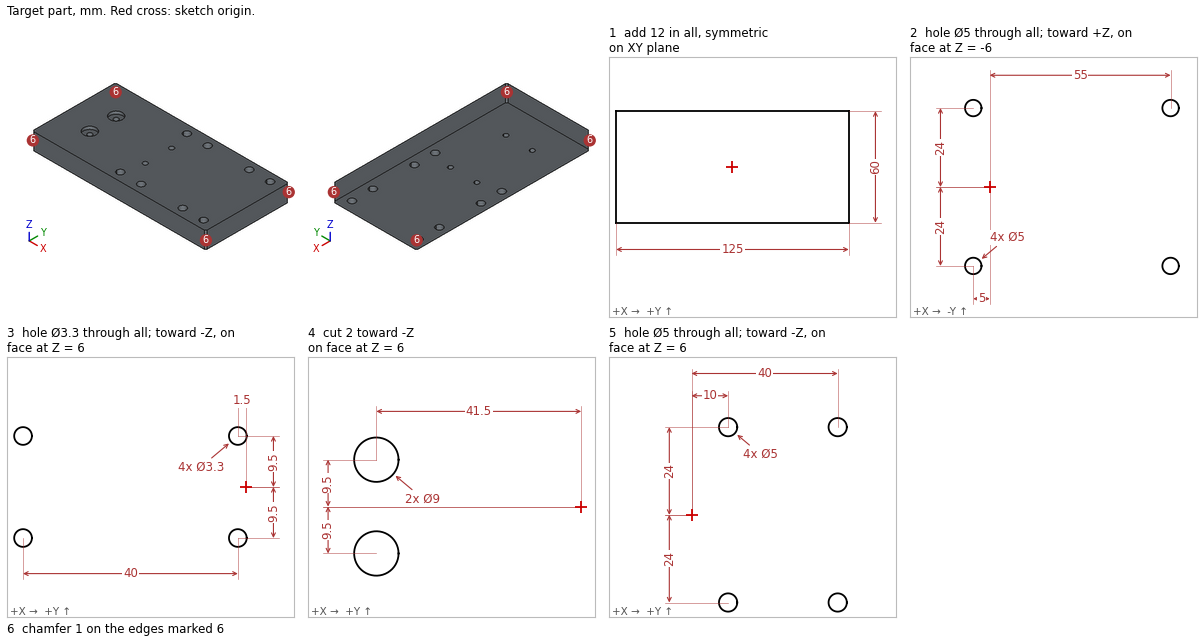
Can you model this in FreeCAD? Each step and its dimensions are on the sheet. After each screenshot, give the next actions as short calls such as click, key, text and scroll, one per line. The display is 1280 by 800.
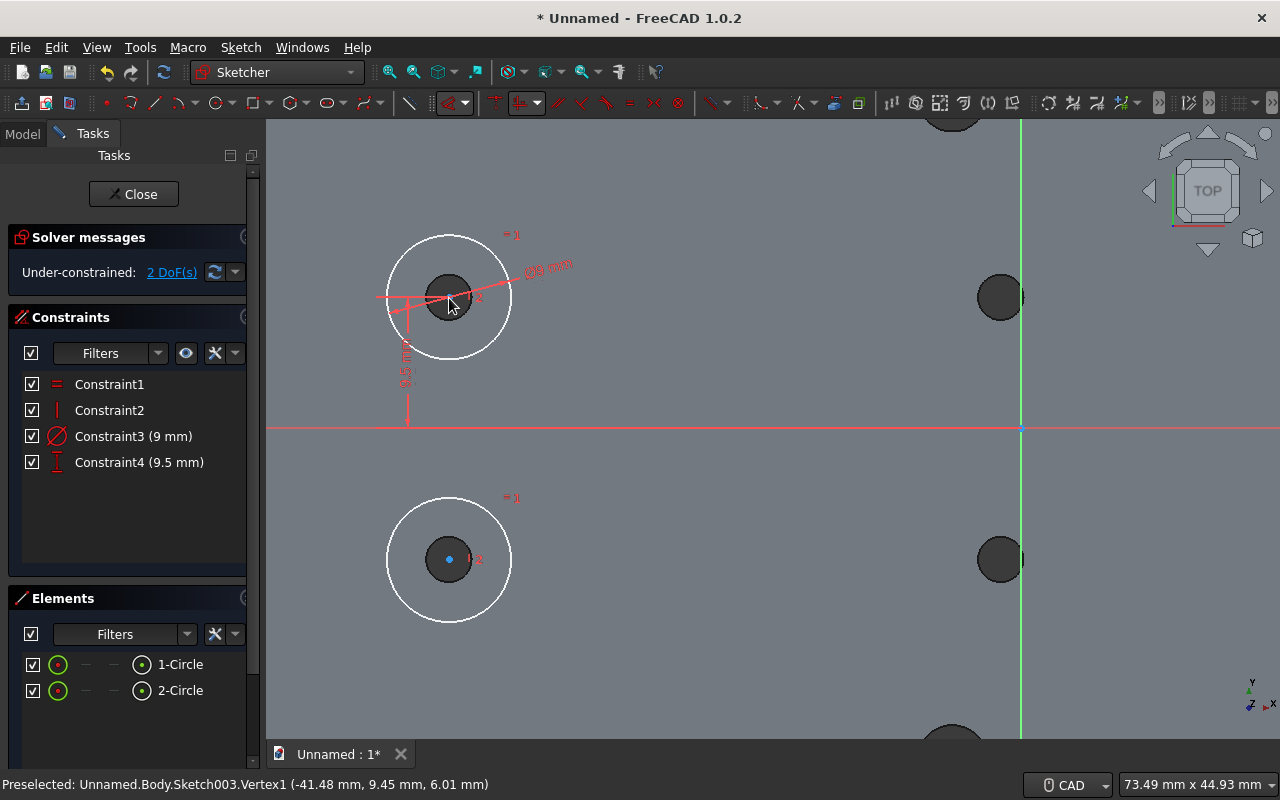
click(449, 560)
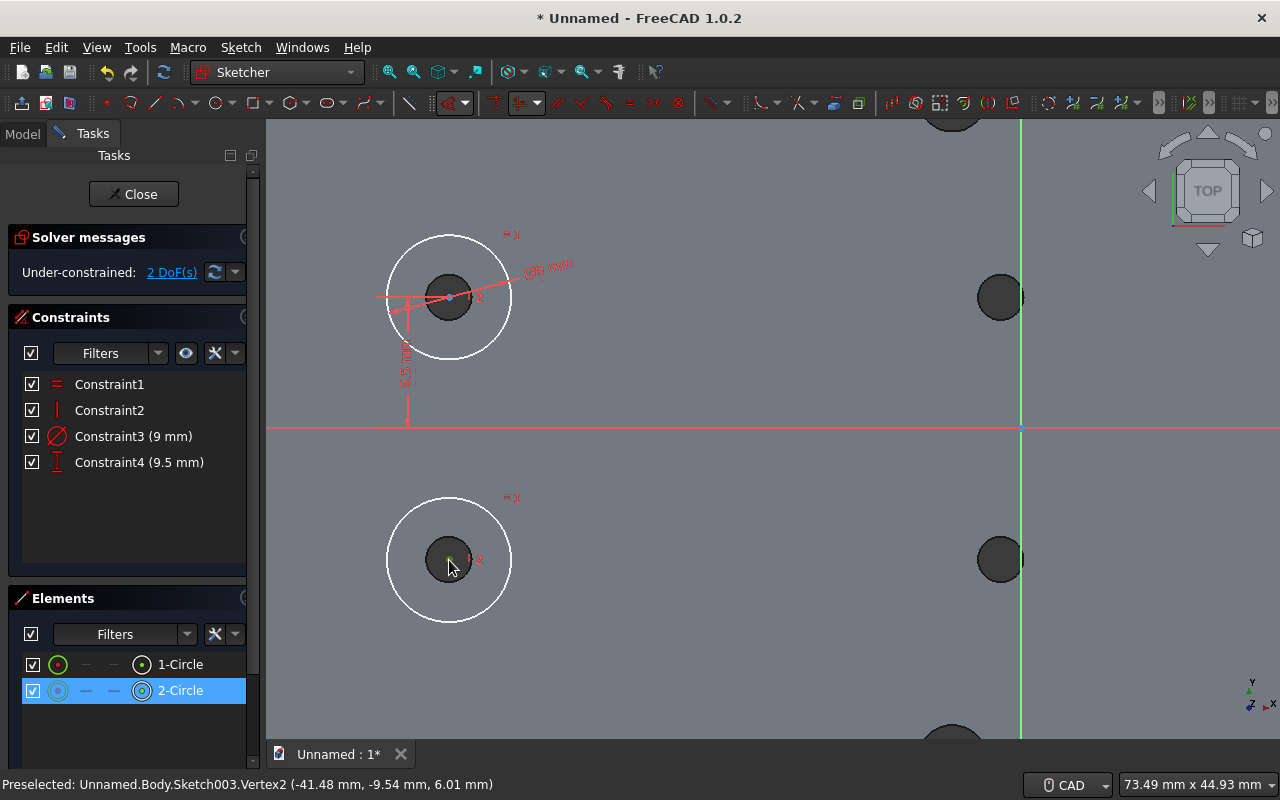
key(i)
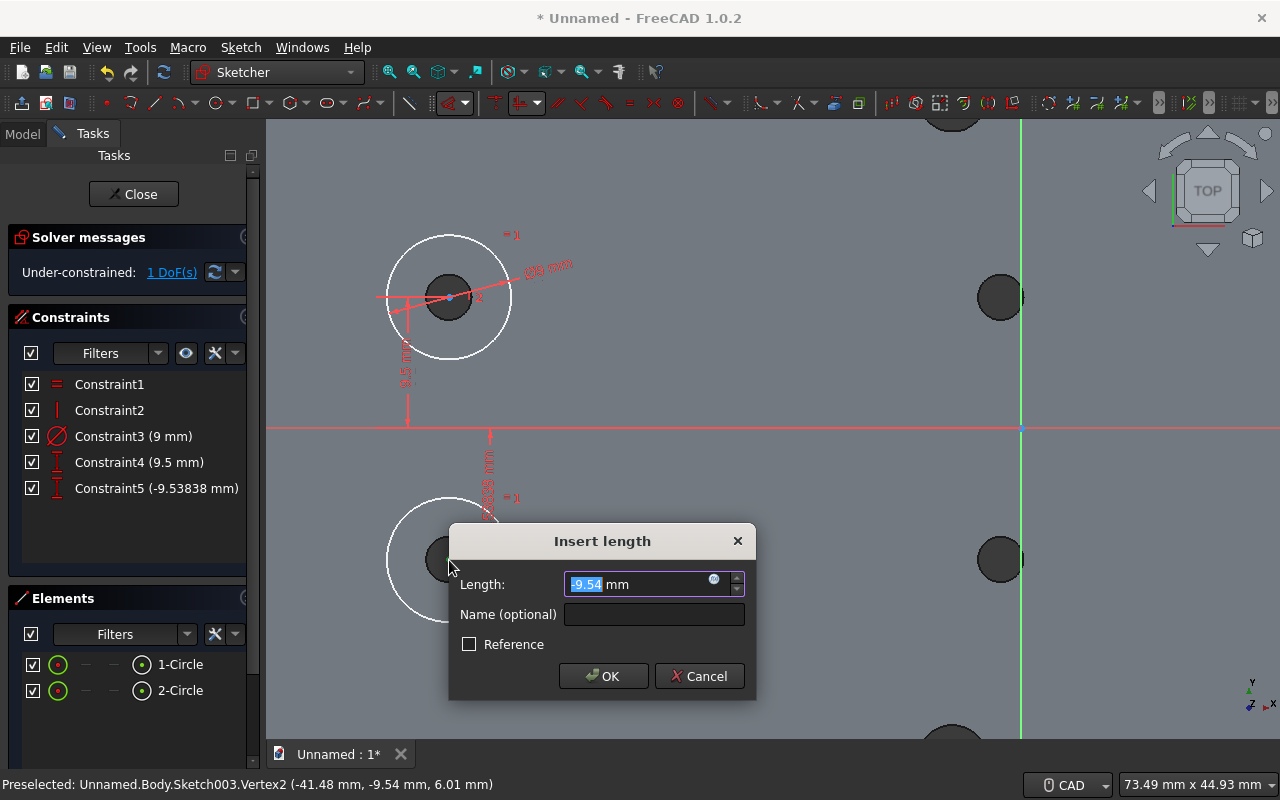
text(-9.5)
key(Return)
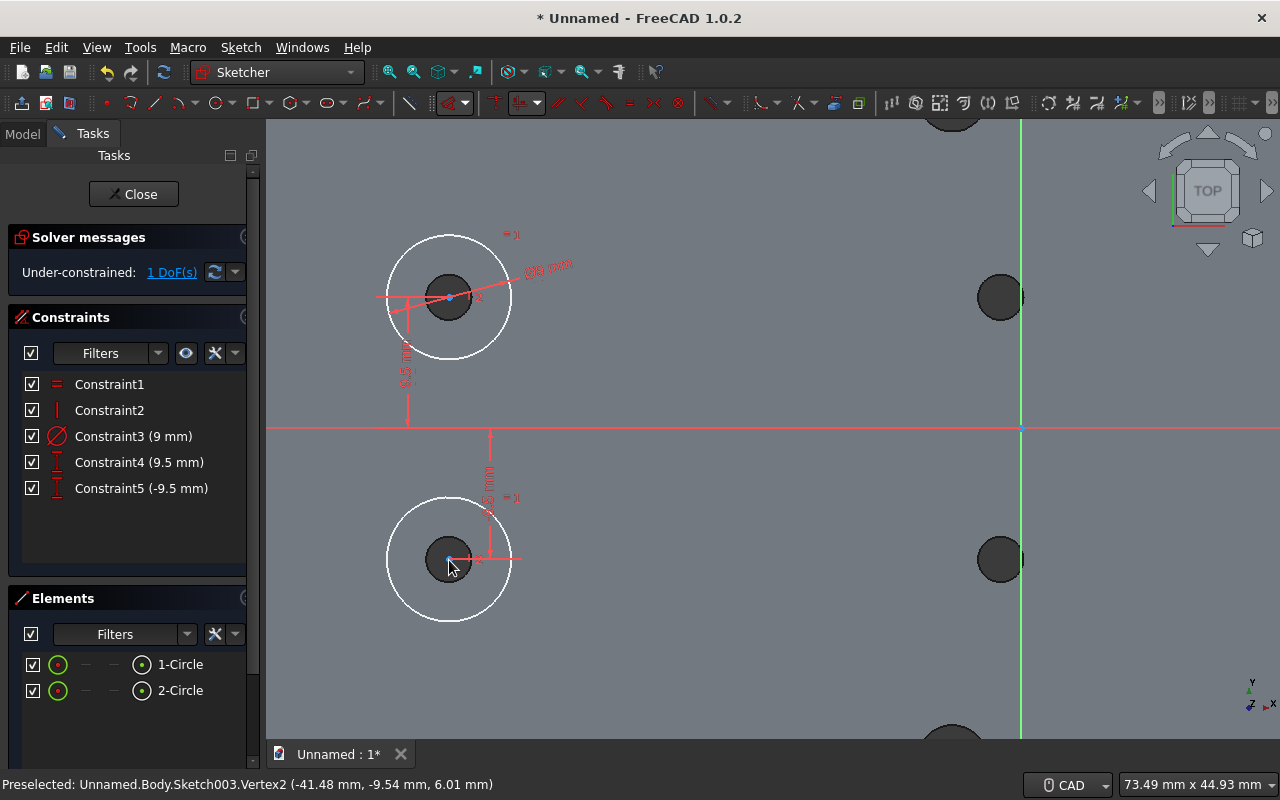
click(449, 297)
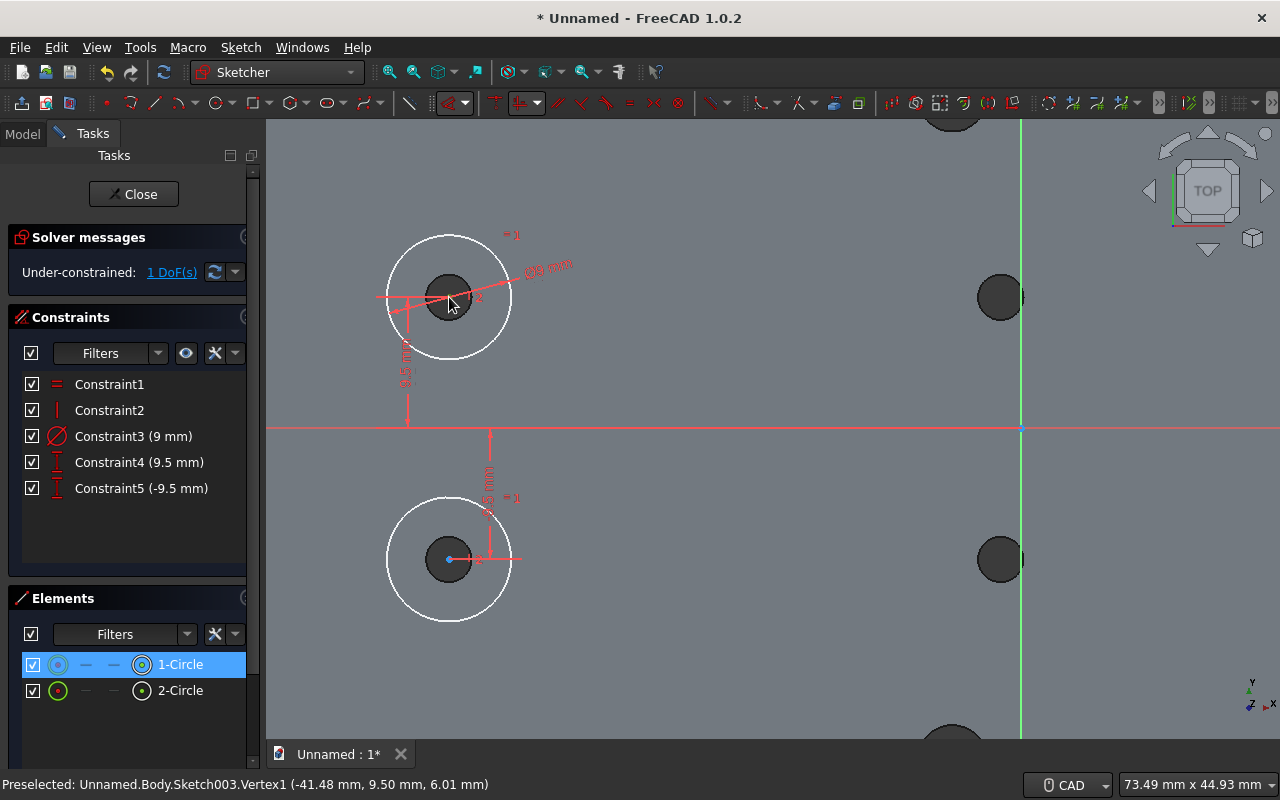
key(l)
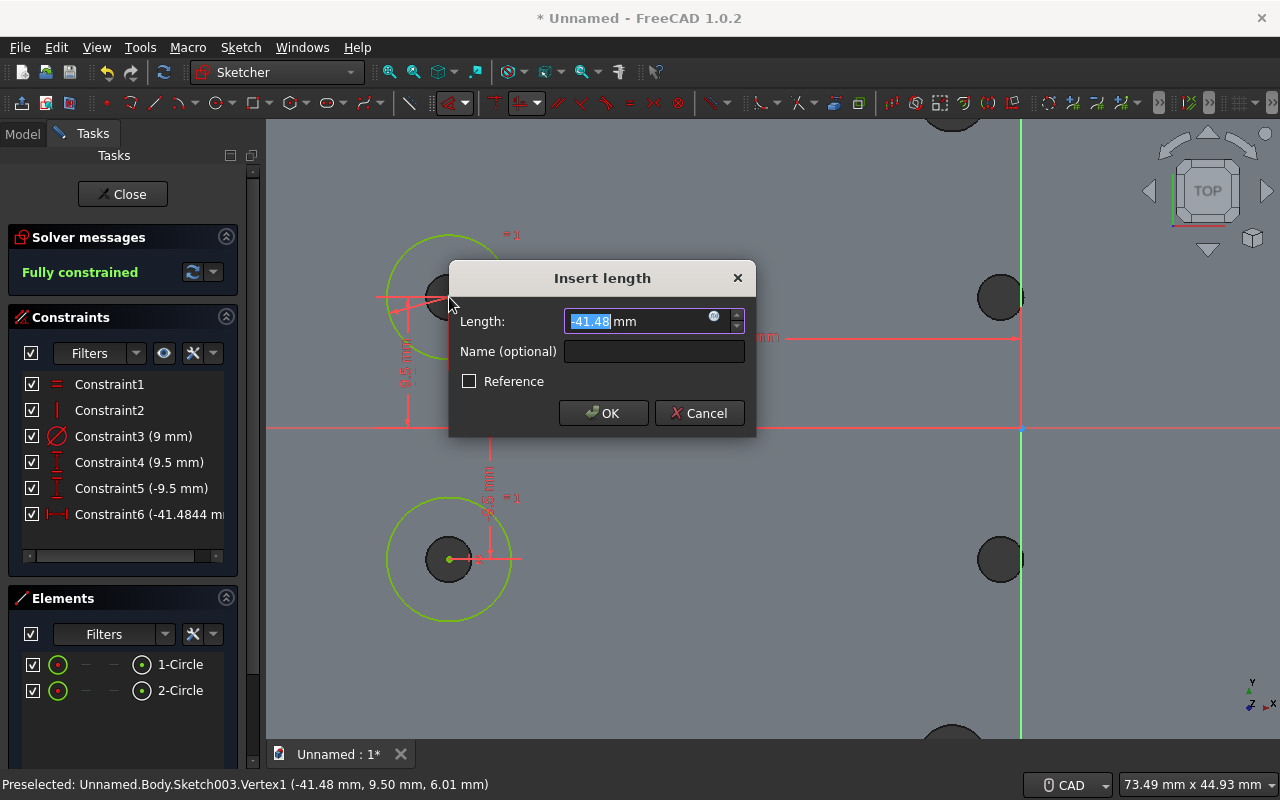
text(-41.5)
key(Return)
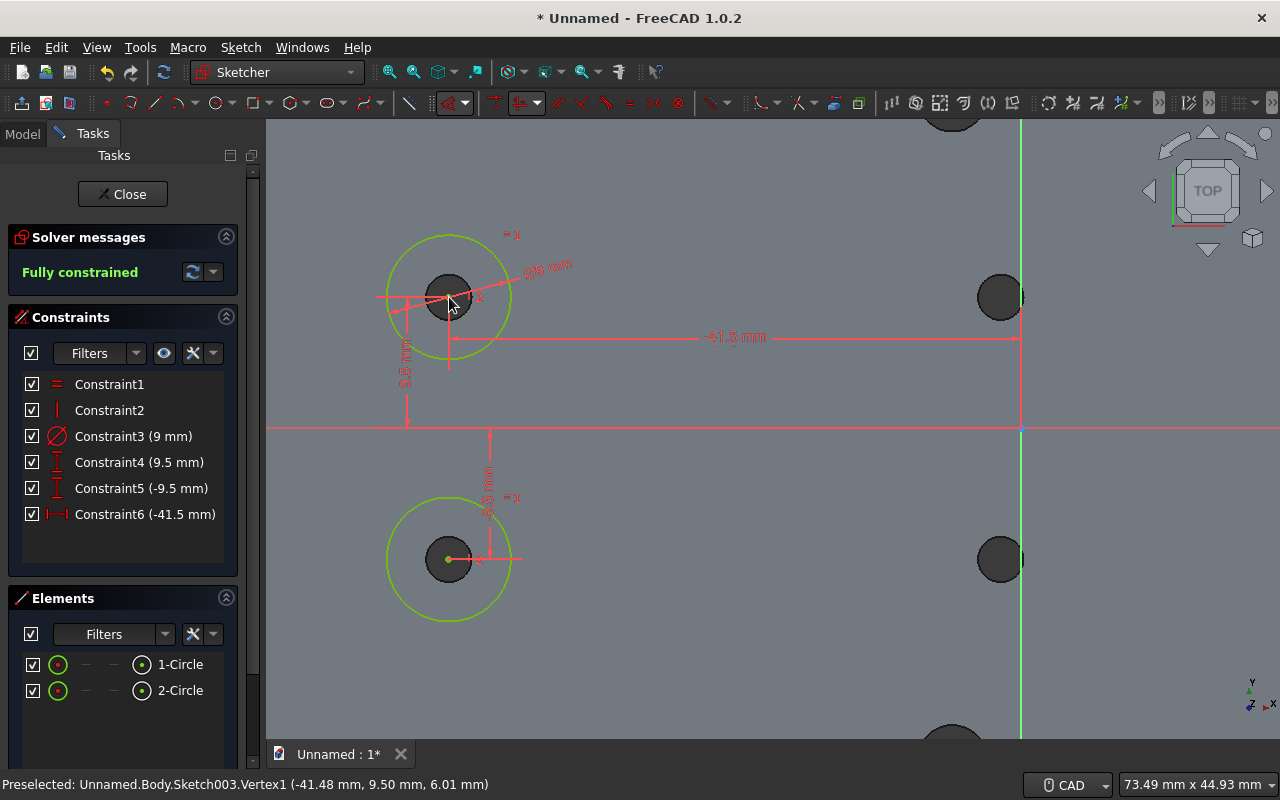
click(123, 194)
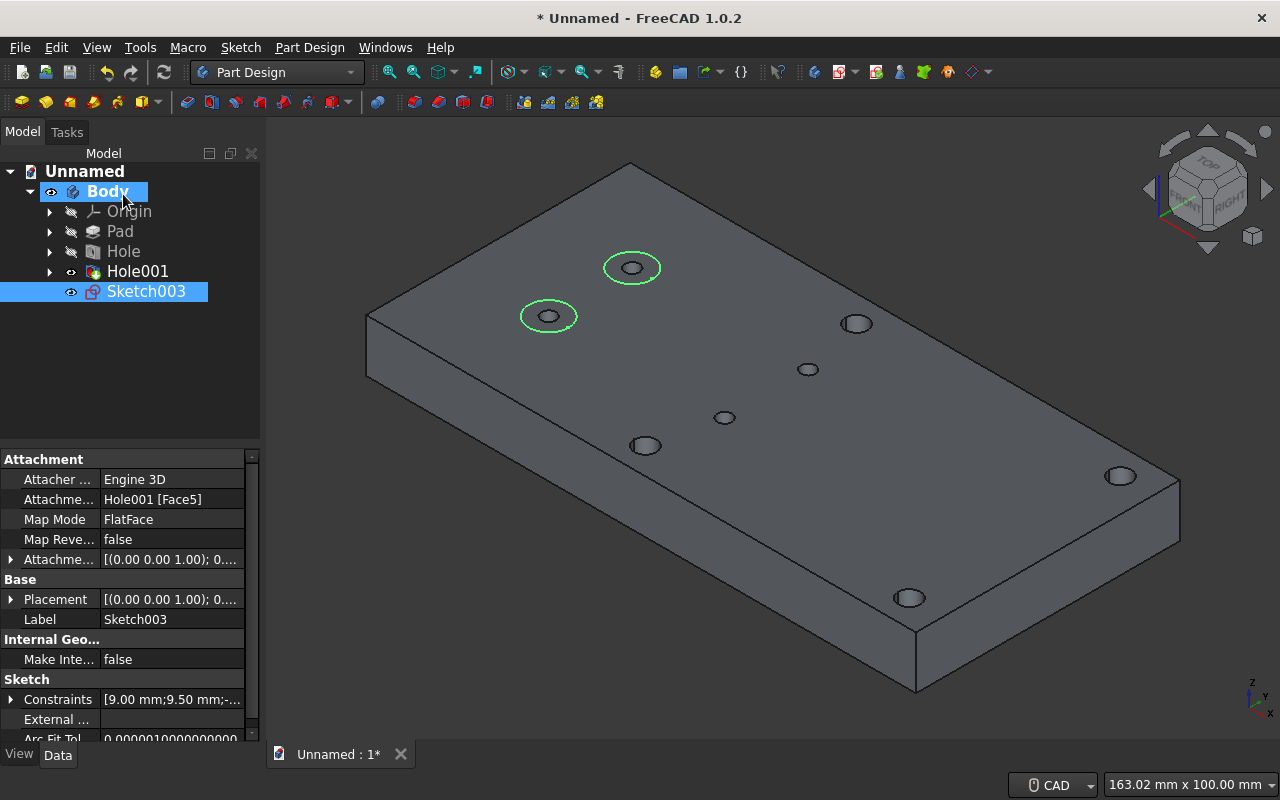
click(188, 102)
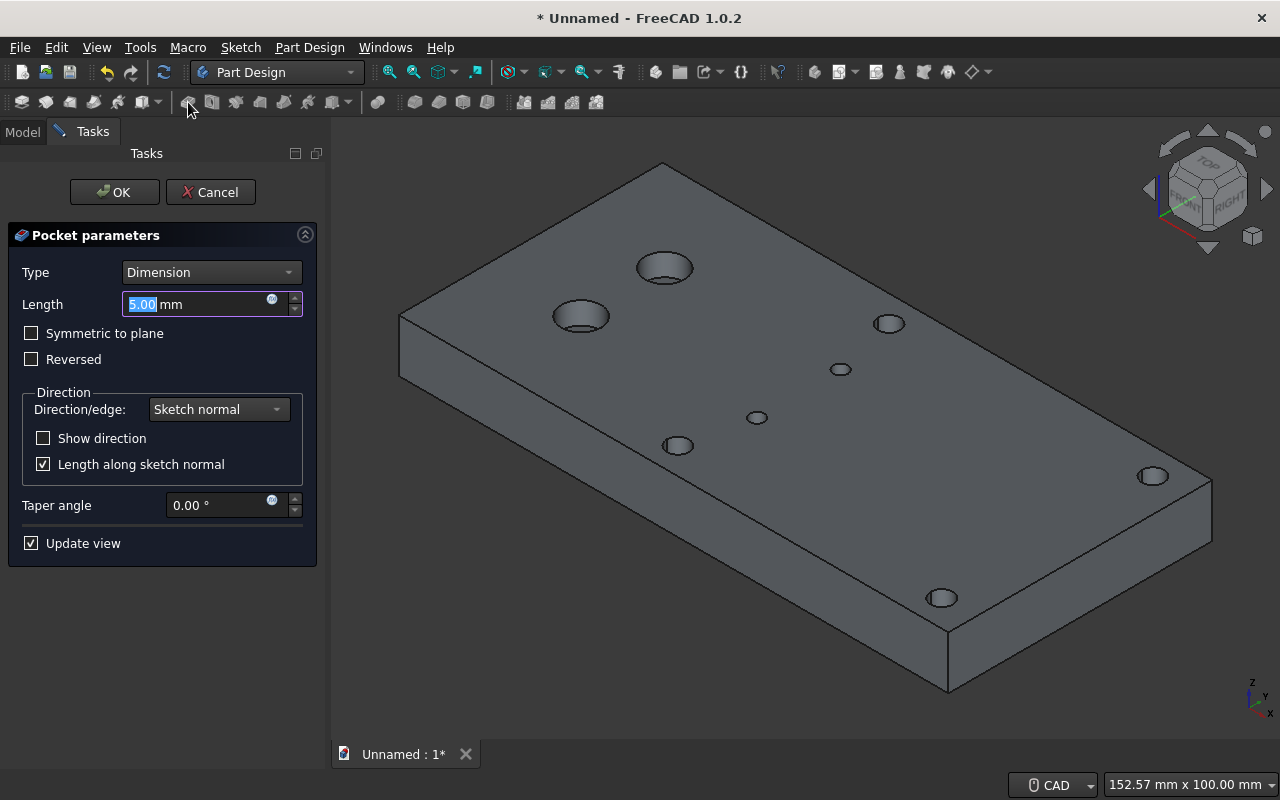
text(2)
key(Tab)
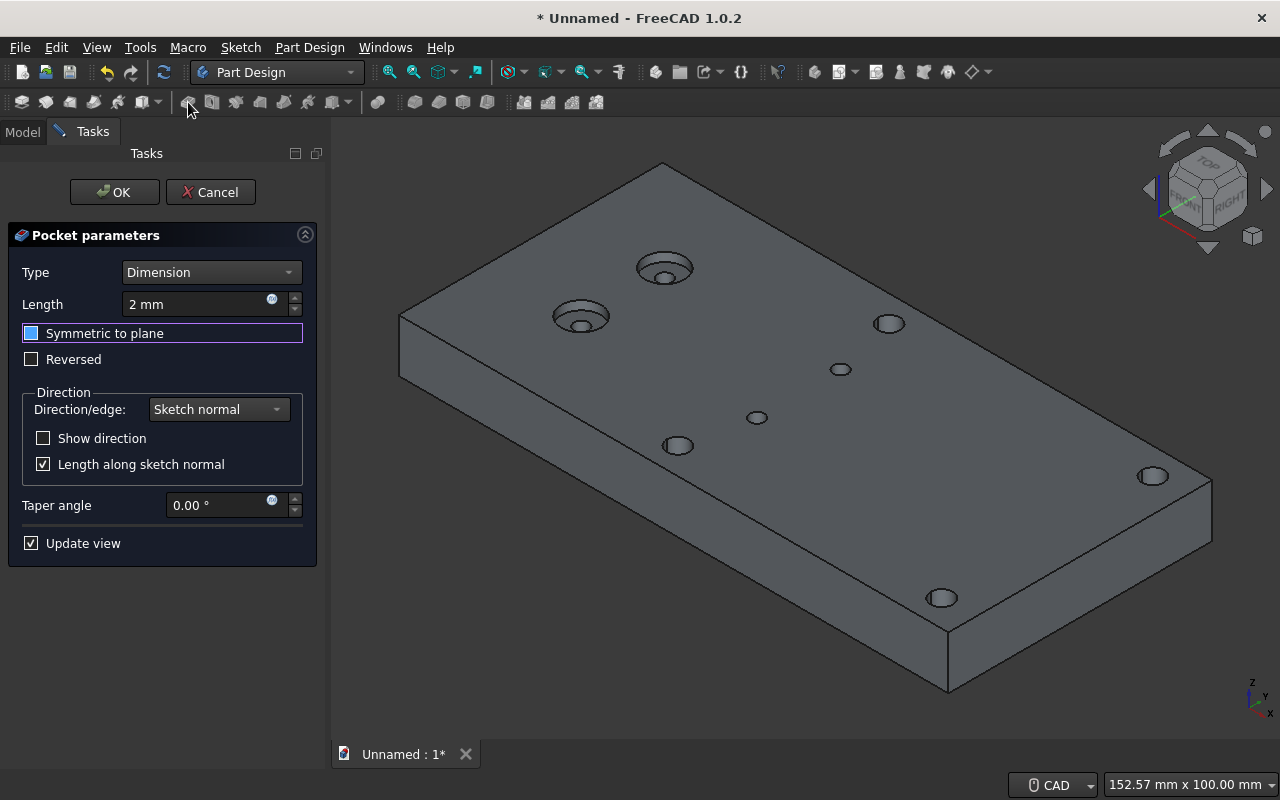
click(115, 192)